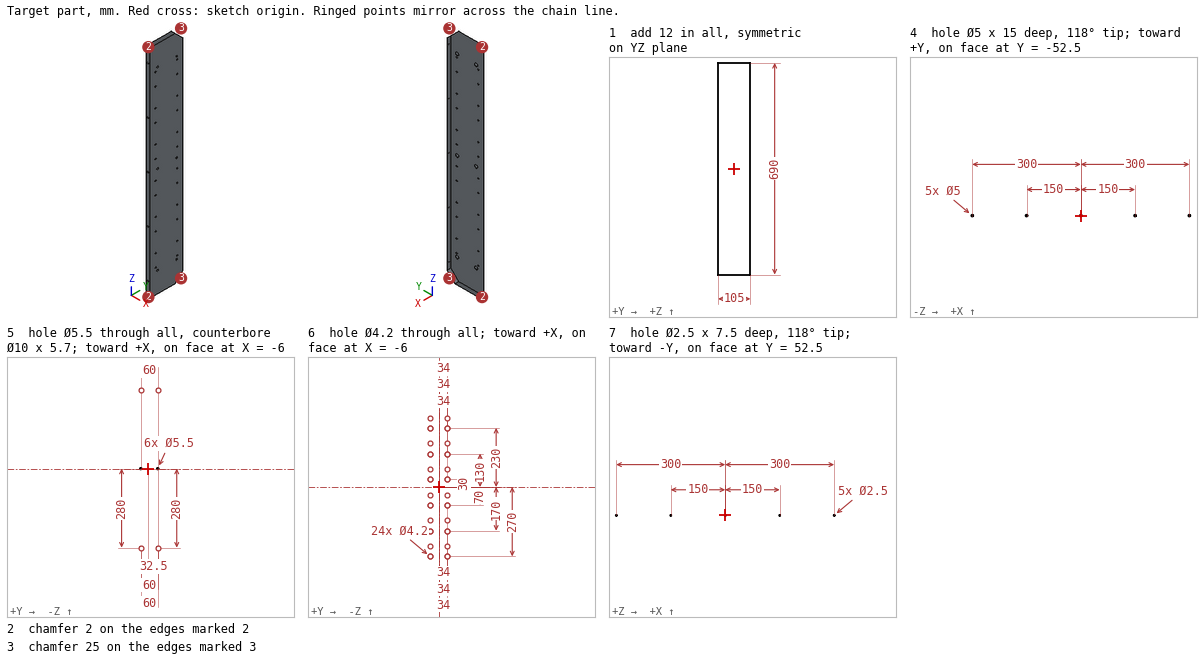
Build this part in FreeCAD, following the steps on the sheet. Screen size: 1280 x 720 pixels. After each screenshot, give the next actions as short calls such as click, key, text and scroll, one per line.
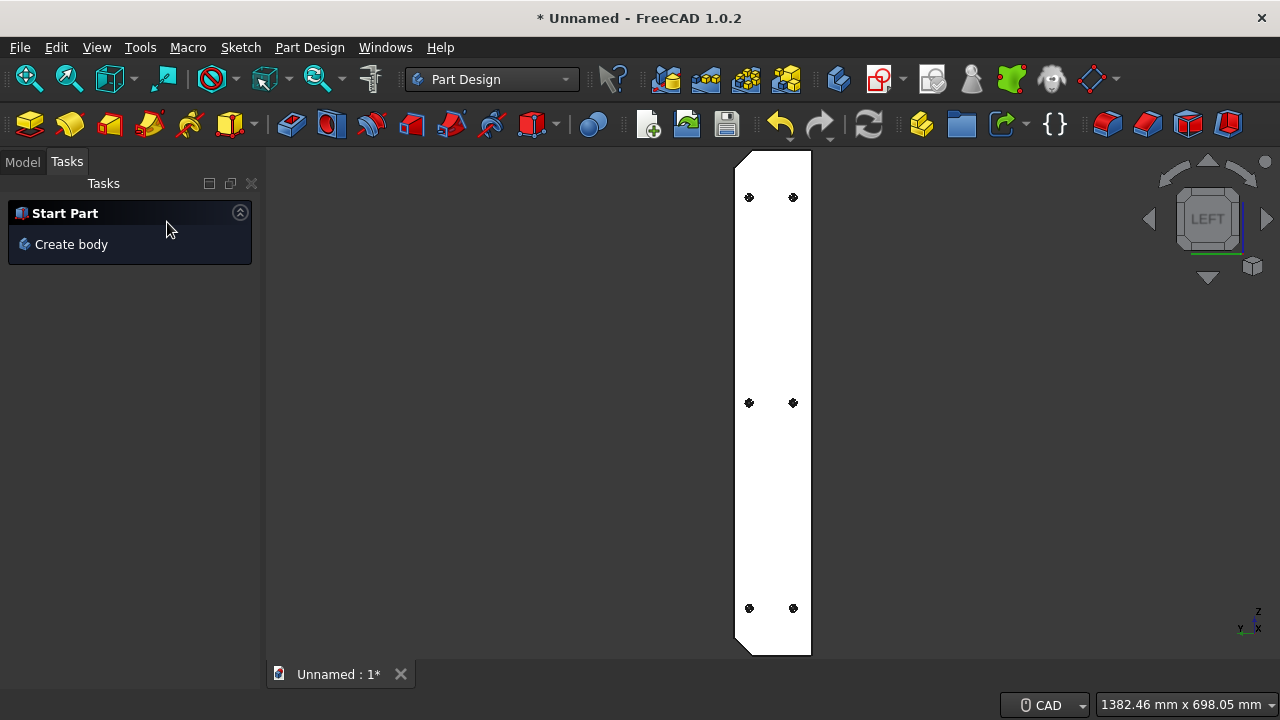
click(773, 547)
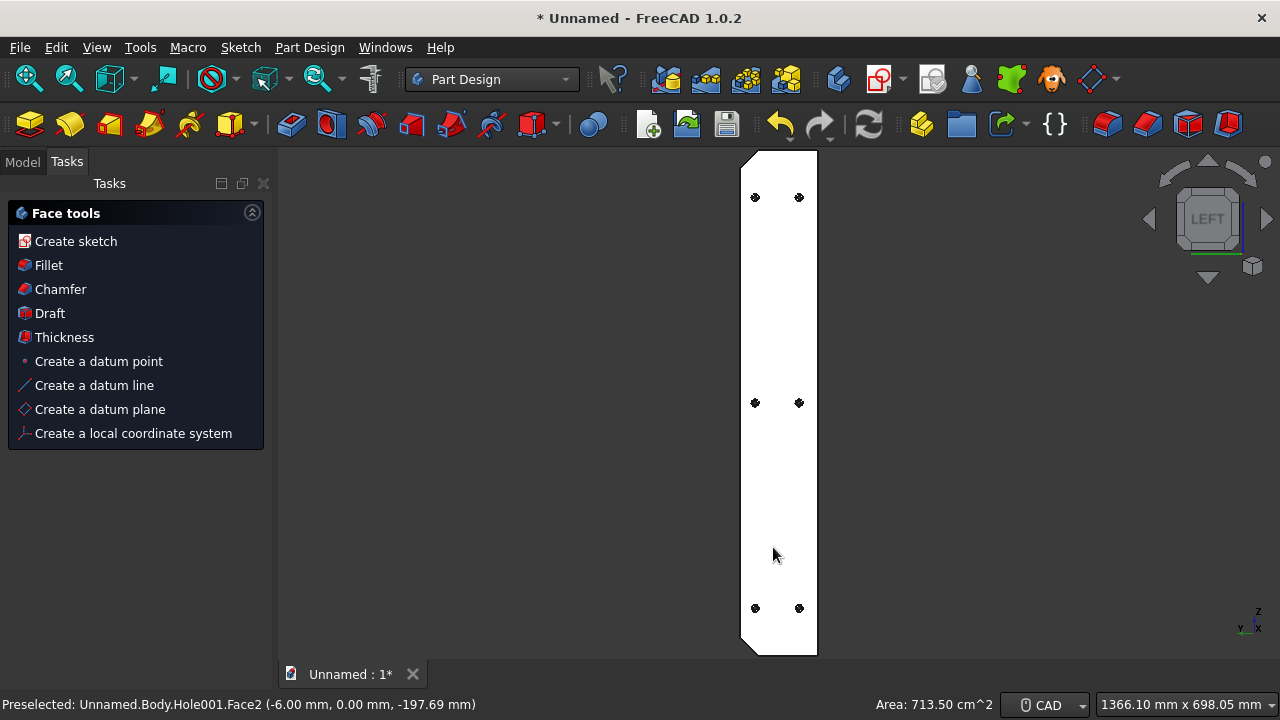
click(880, 80)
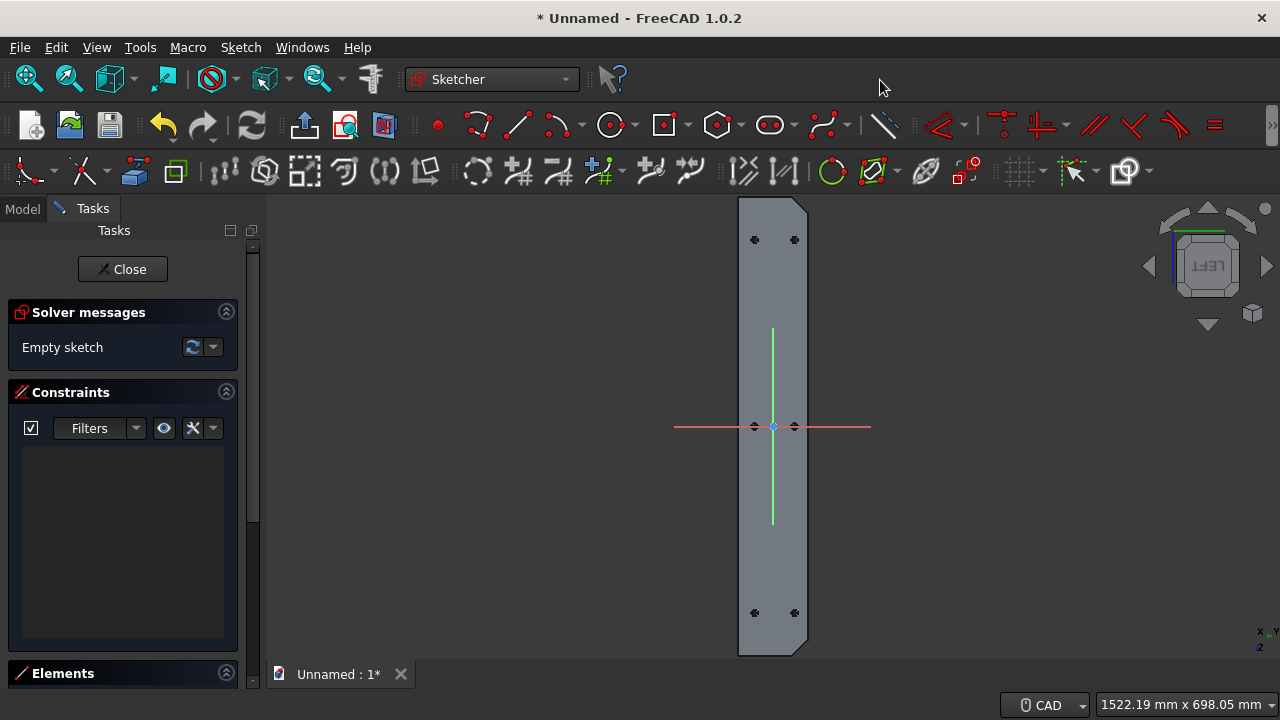
scroll(395, 427, down, 1)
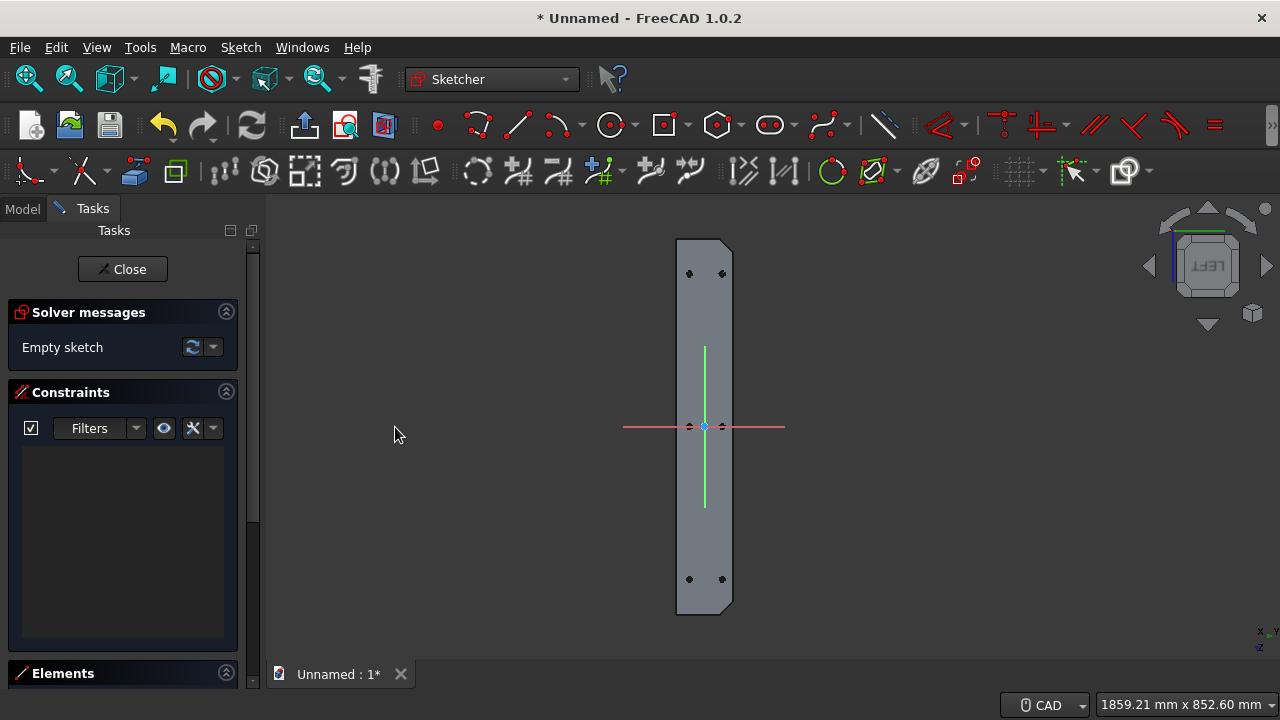
click(612, 126)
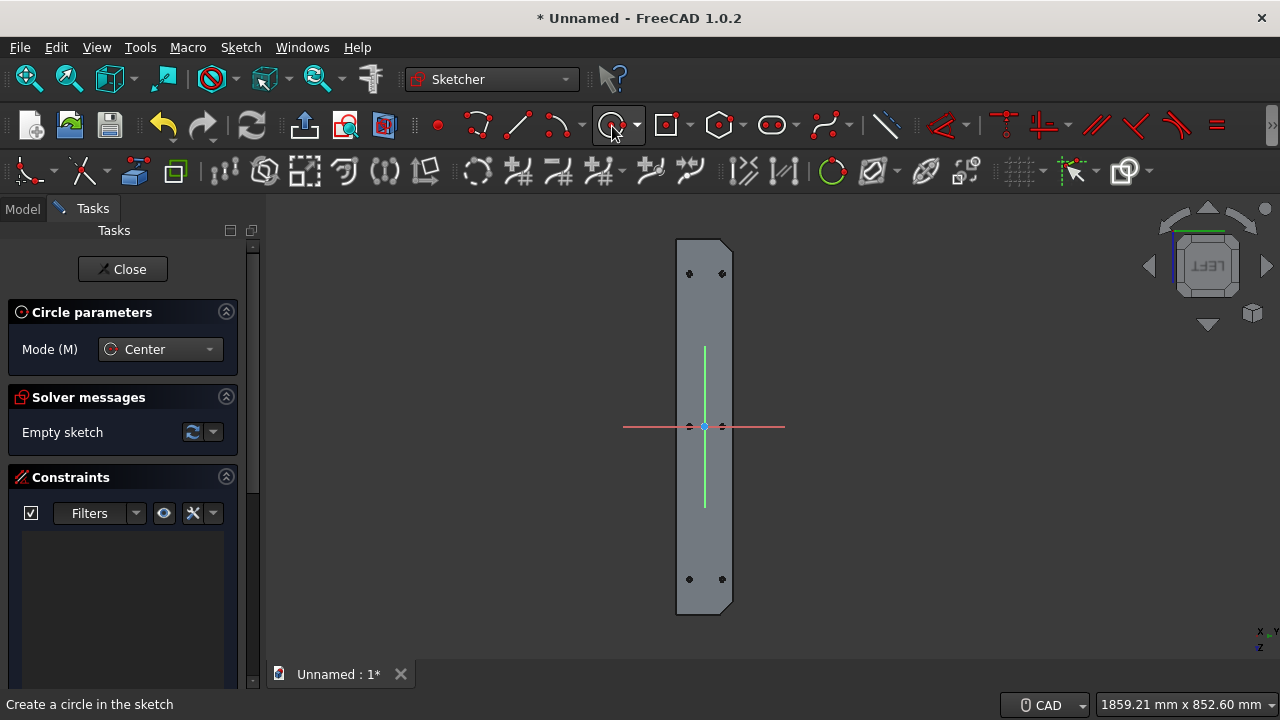
scroll(723, 574, up, 15)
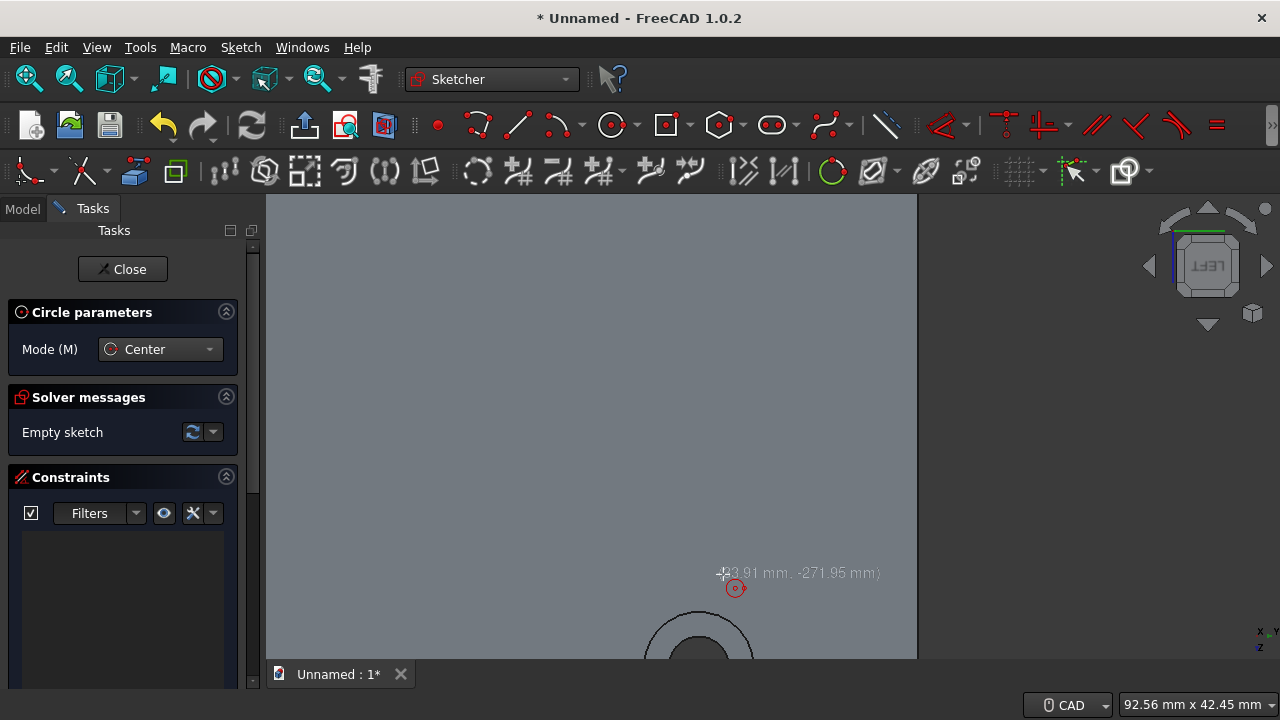
scroll(723, 575, down, 15)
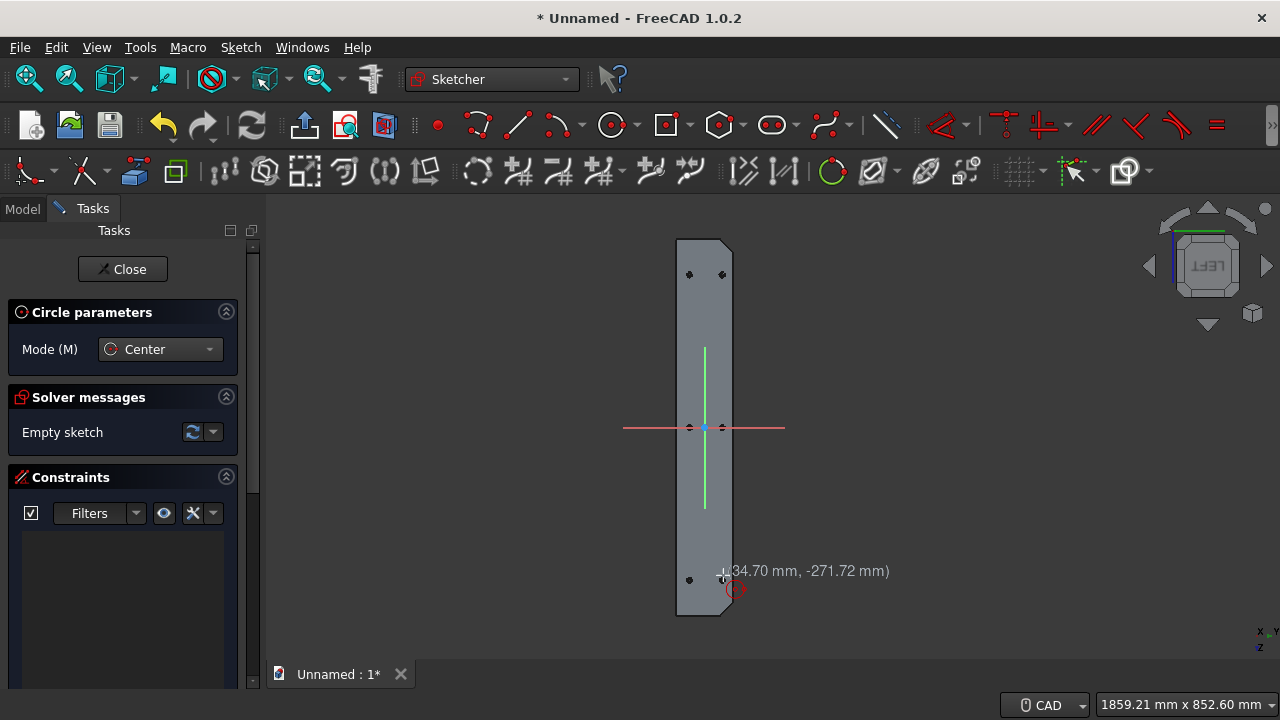
click(723, 575)
move(724, 574)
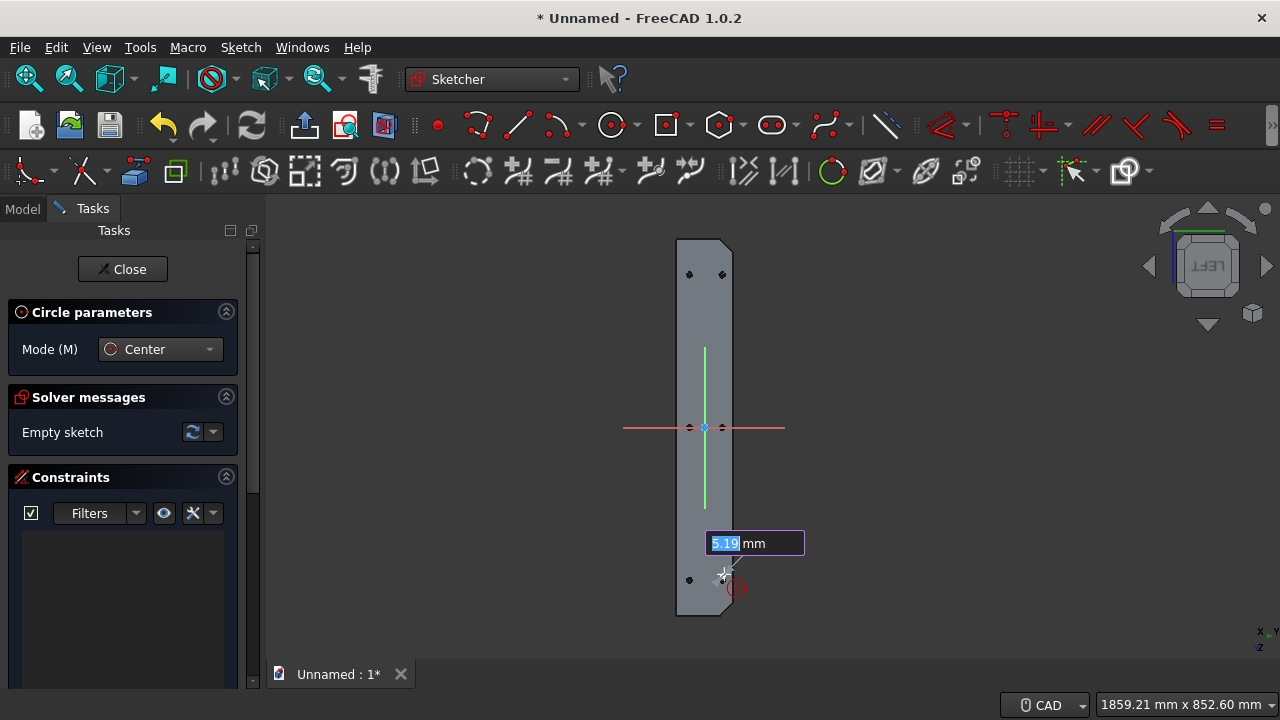
text(4.2)
key(Return)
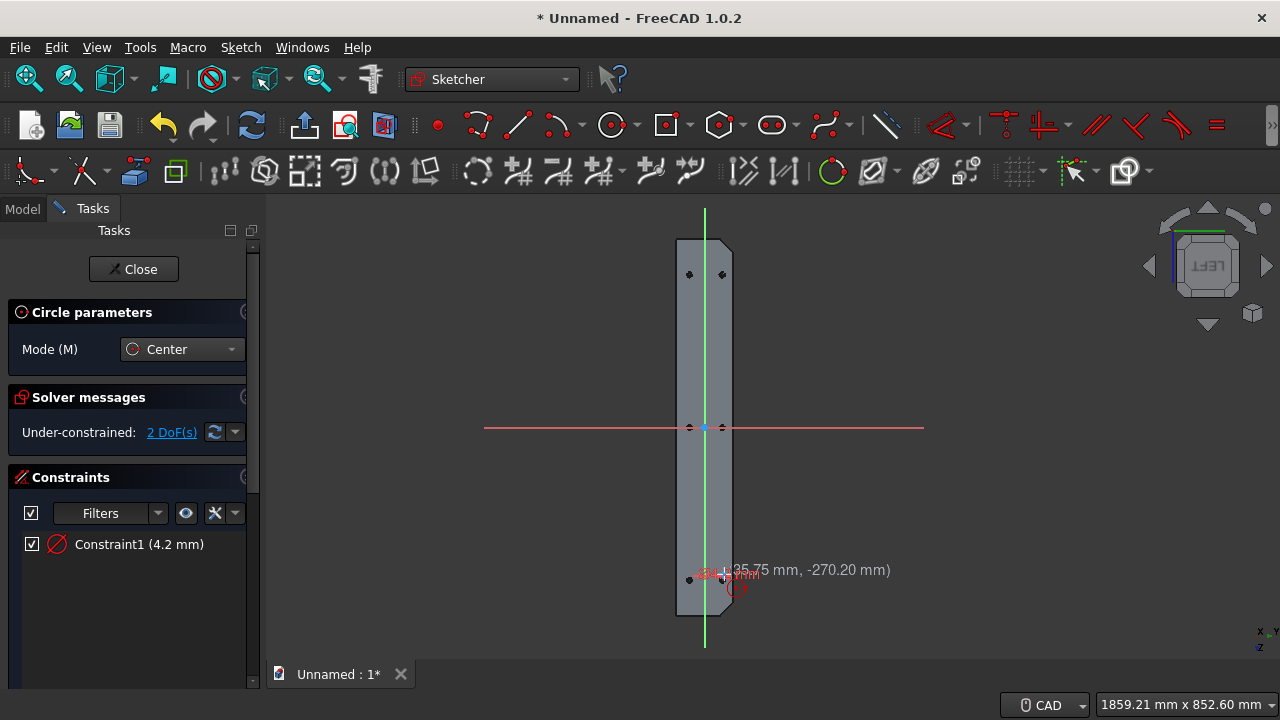
scroll(686, 575, up, 15)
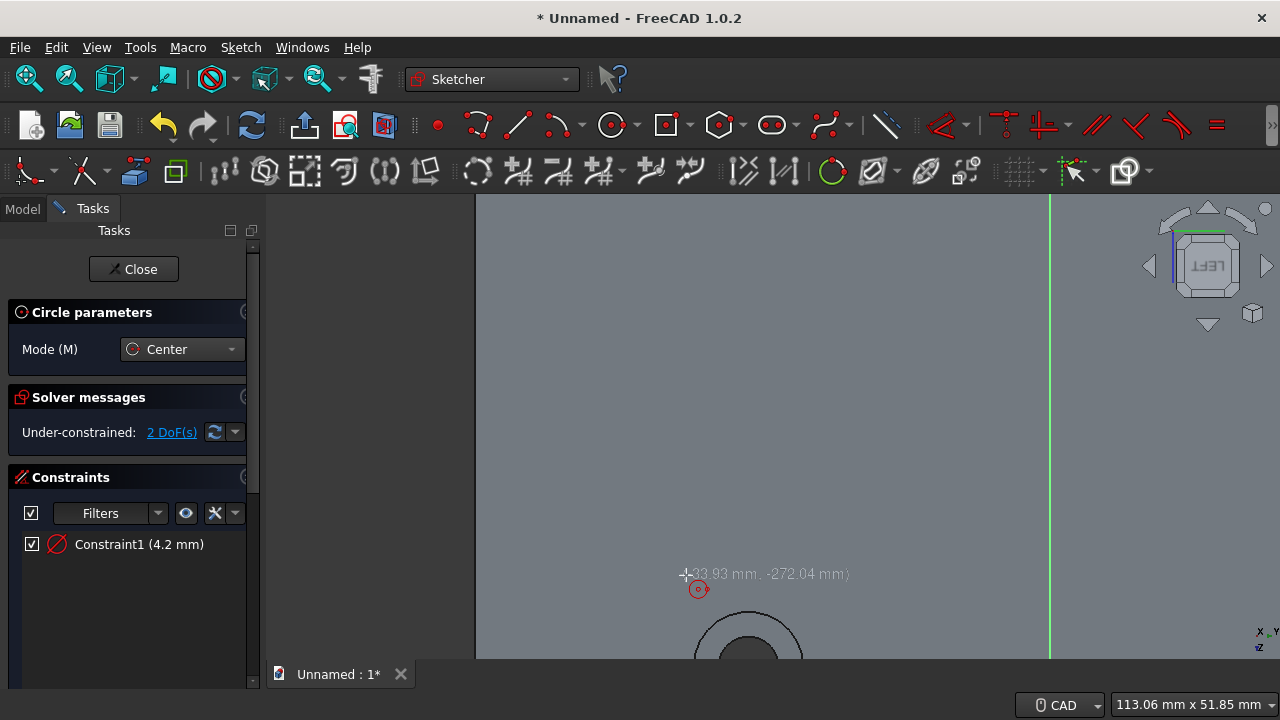
scroll(686, 575, down, 15)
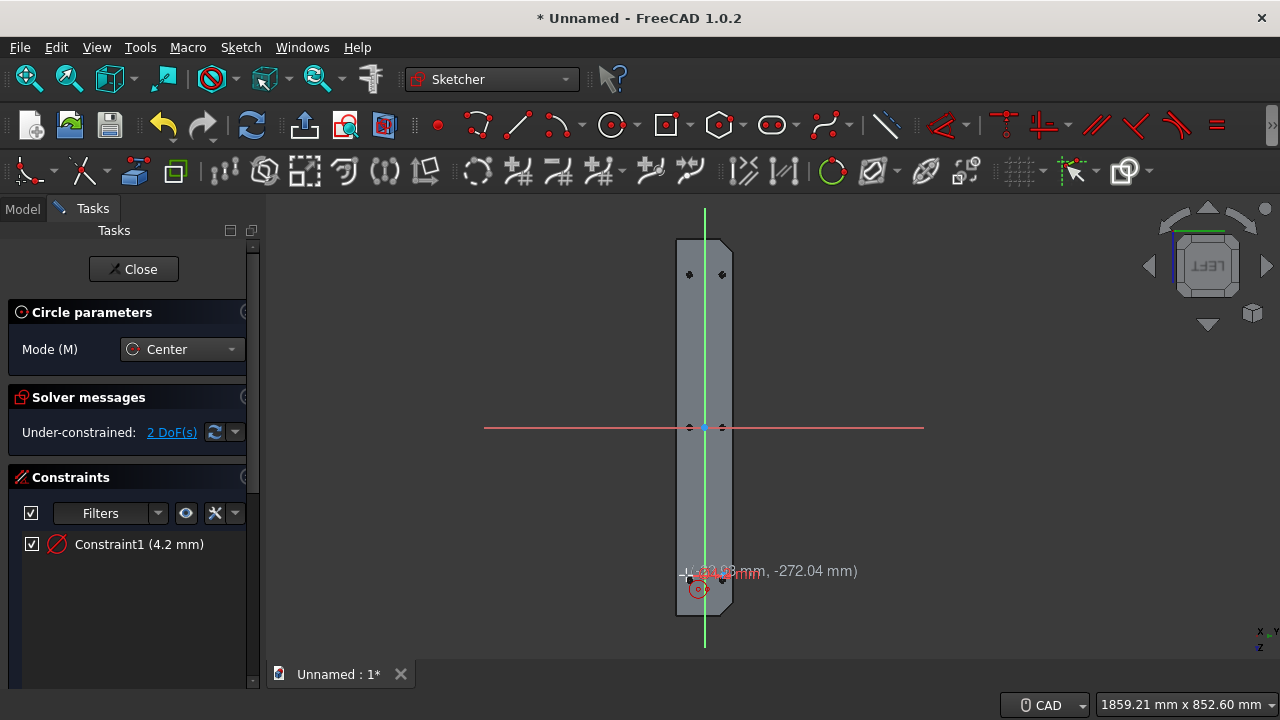
click(686, 575)
move(687, 574)